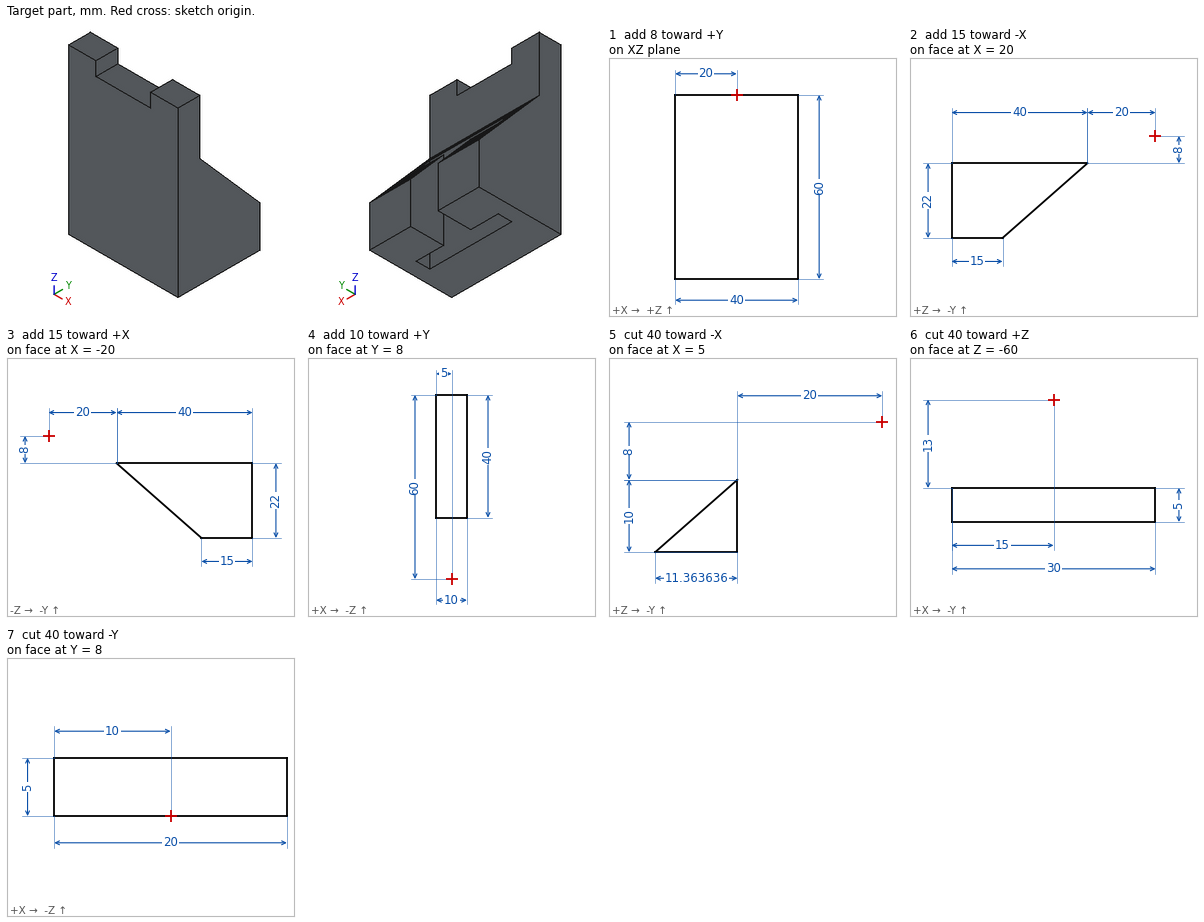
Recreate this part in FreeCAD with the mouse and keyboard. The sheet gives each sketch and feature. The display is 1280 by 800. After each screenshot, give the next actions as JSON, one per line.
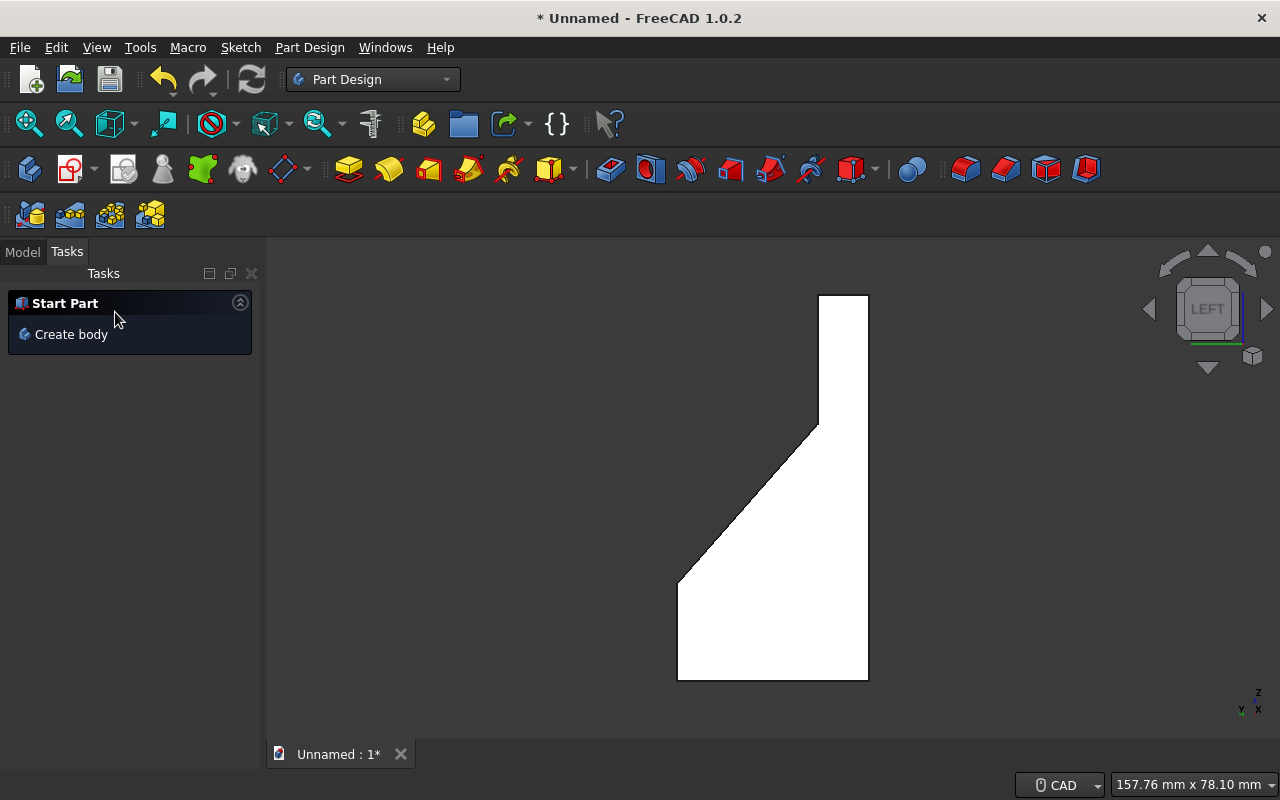
{"action": "key", "text": "4"}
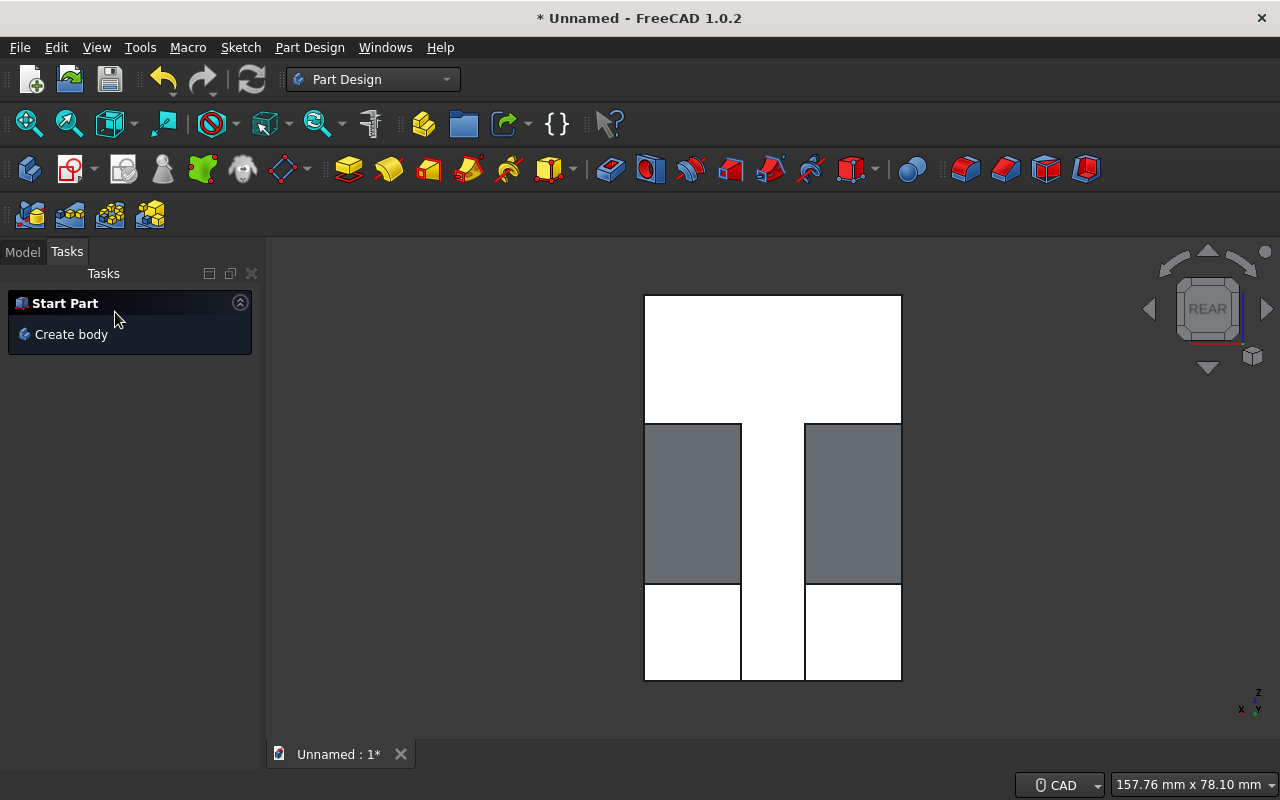
{"action": "left_click", "coordinate": [773, 377]}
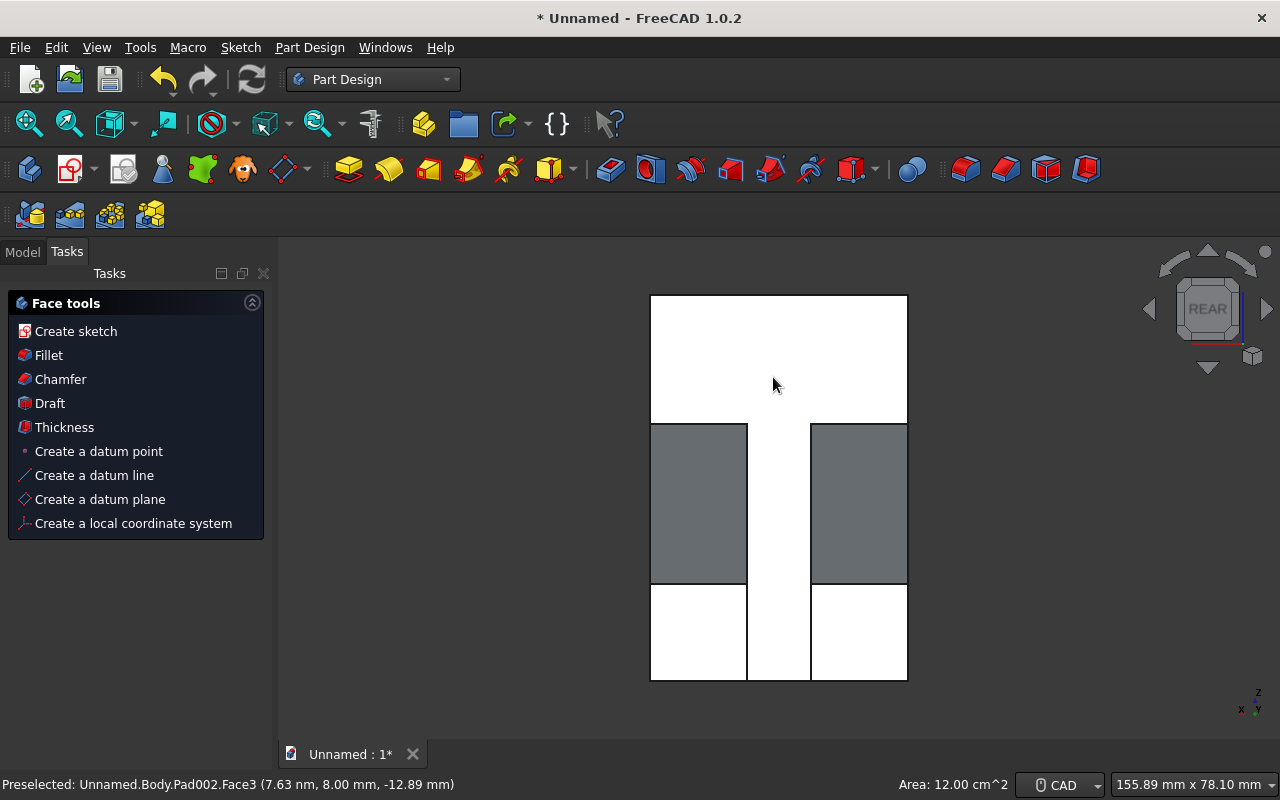
{"action": "left_click", "coordinate": [70, 170]}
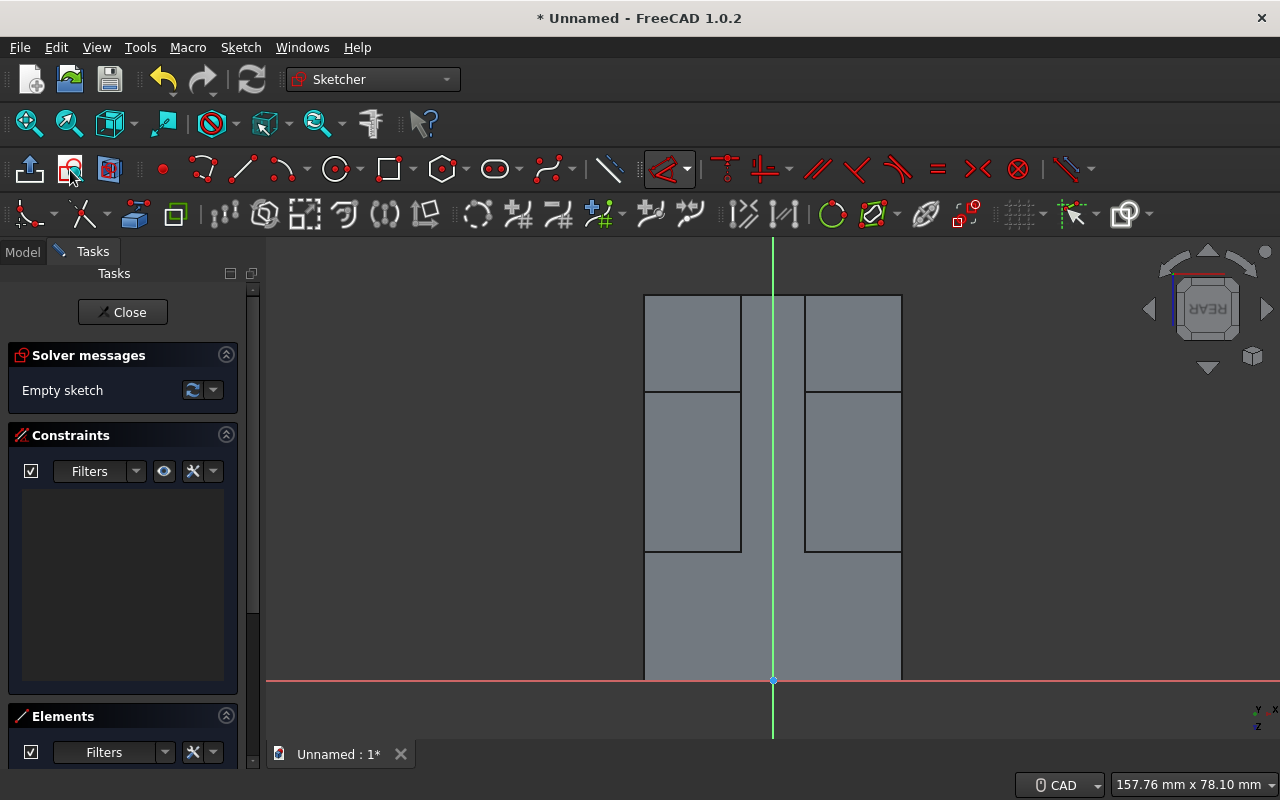
{"action": "left_click", "coordinate": [110, 170]}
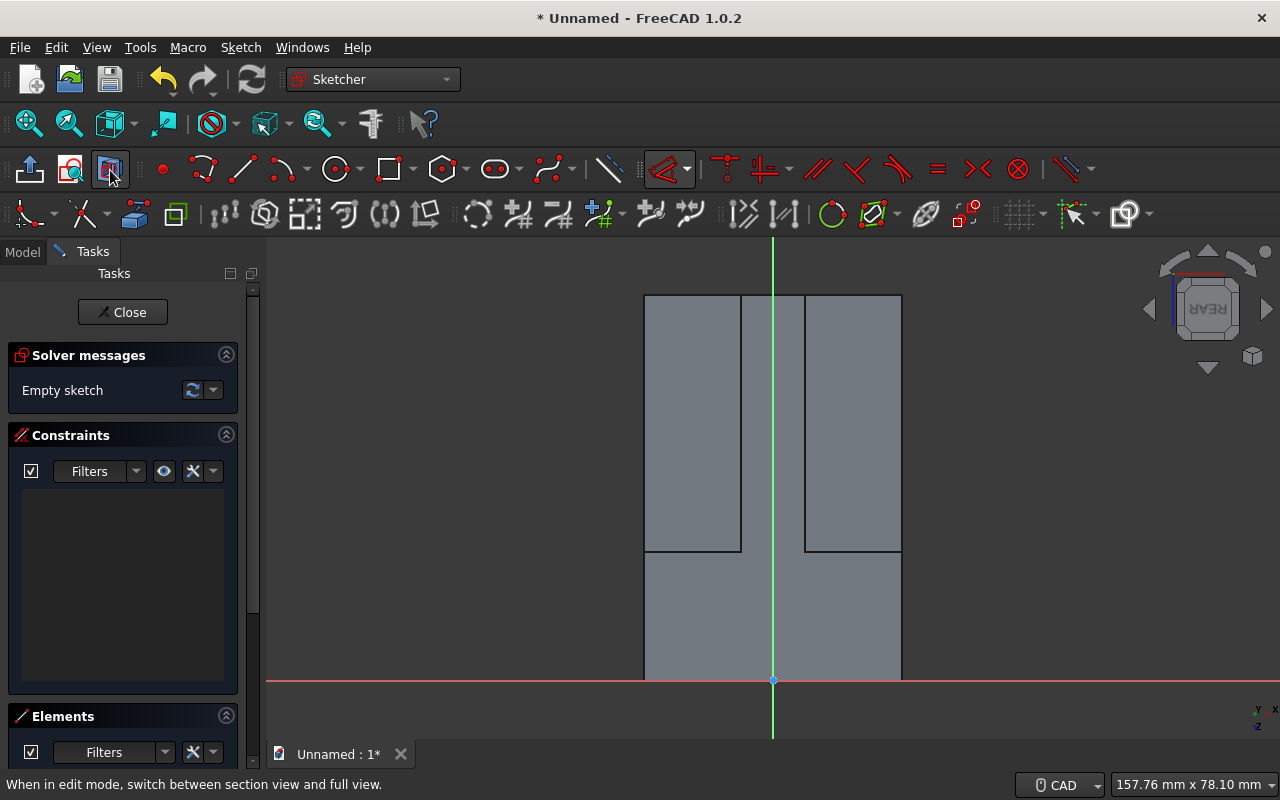
{"action": "left_click", "coordinate": [390, 170]}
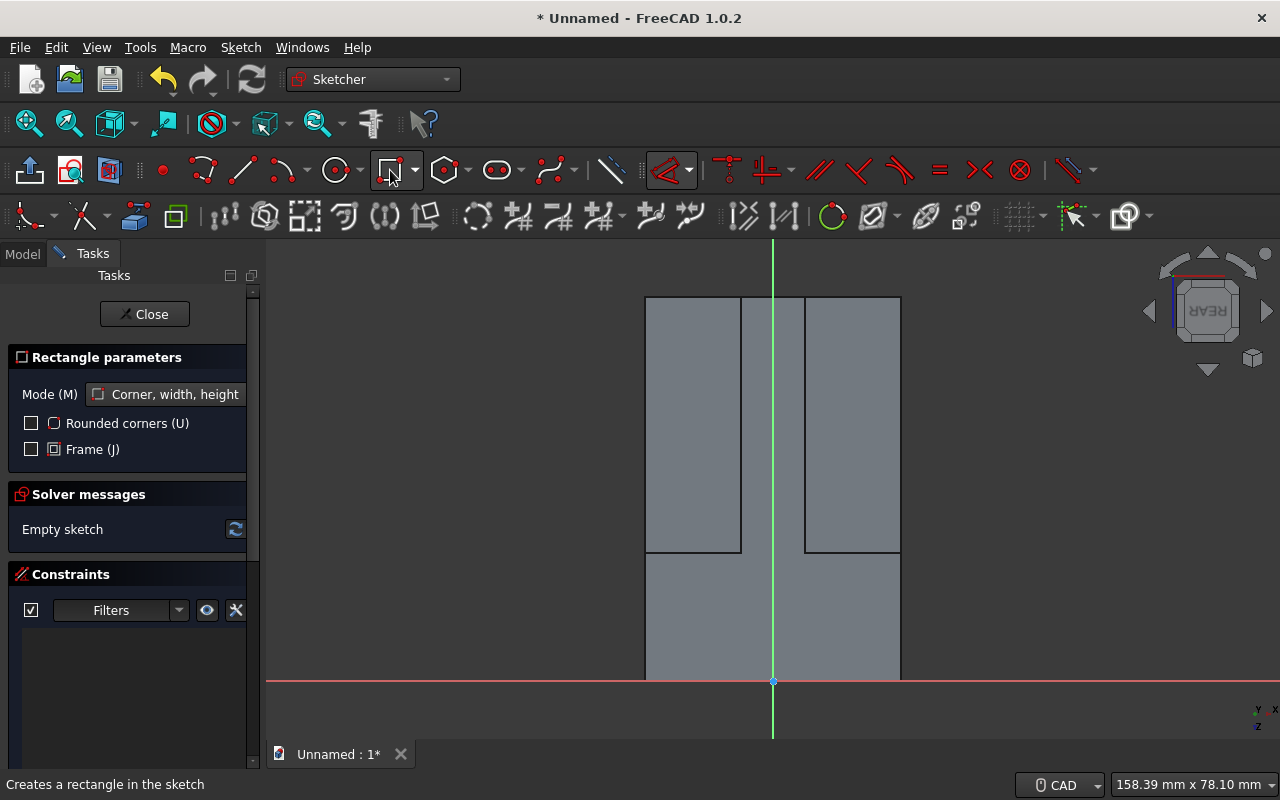
{"action": "left_click", "coordinate": [741, 297]}
{"action": "mouse_move", "coordinate": [805, 553]}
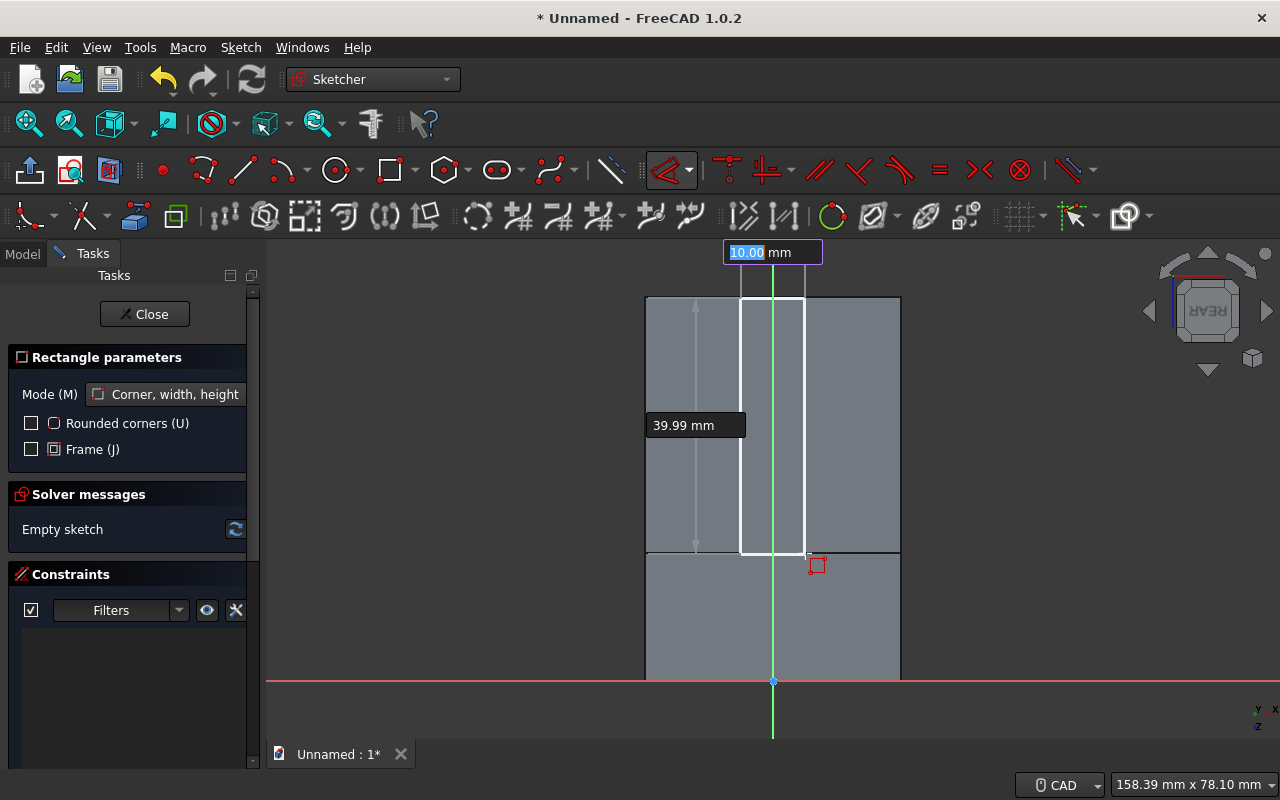
{"action": "type", "text": "10"}
{"action": "key", "text": "Tab"}
{"action": "type", "text": "40"}
{"action": "key", "text": "Return"}
{"action": "key", "text": "Escape"}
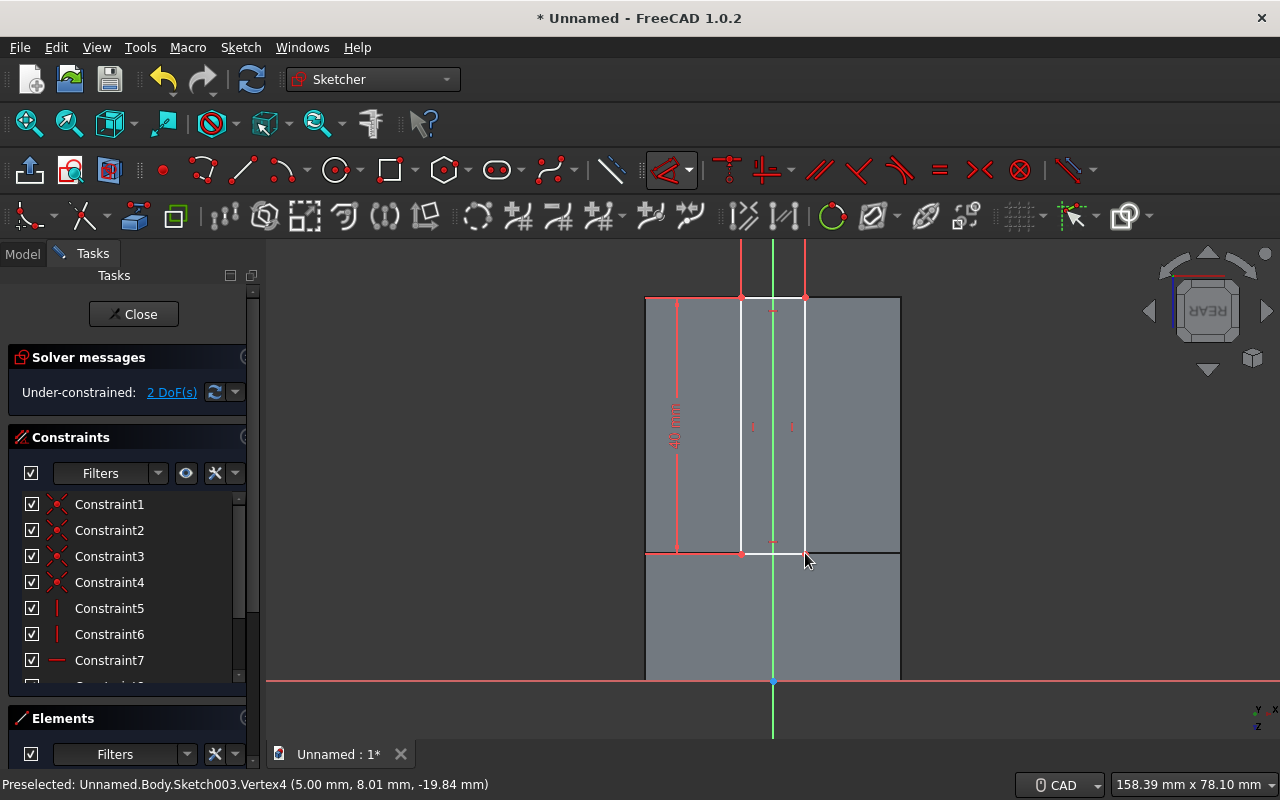
{"action": "scroll", "coordinate": [741, 298], "scroll_direction": "up", "scroll_amount": 2}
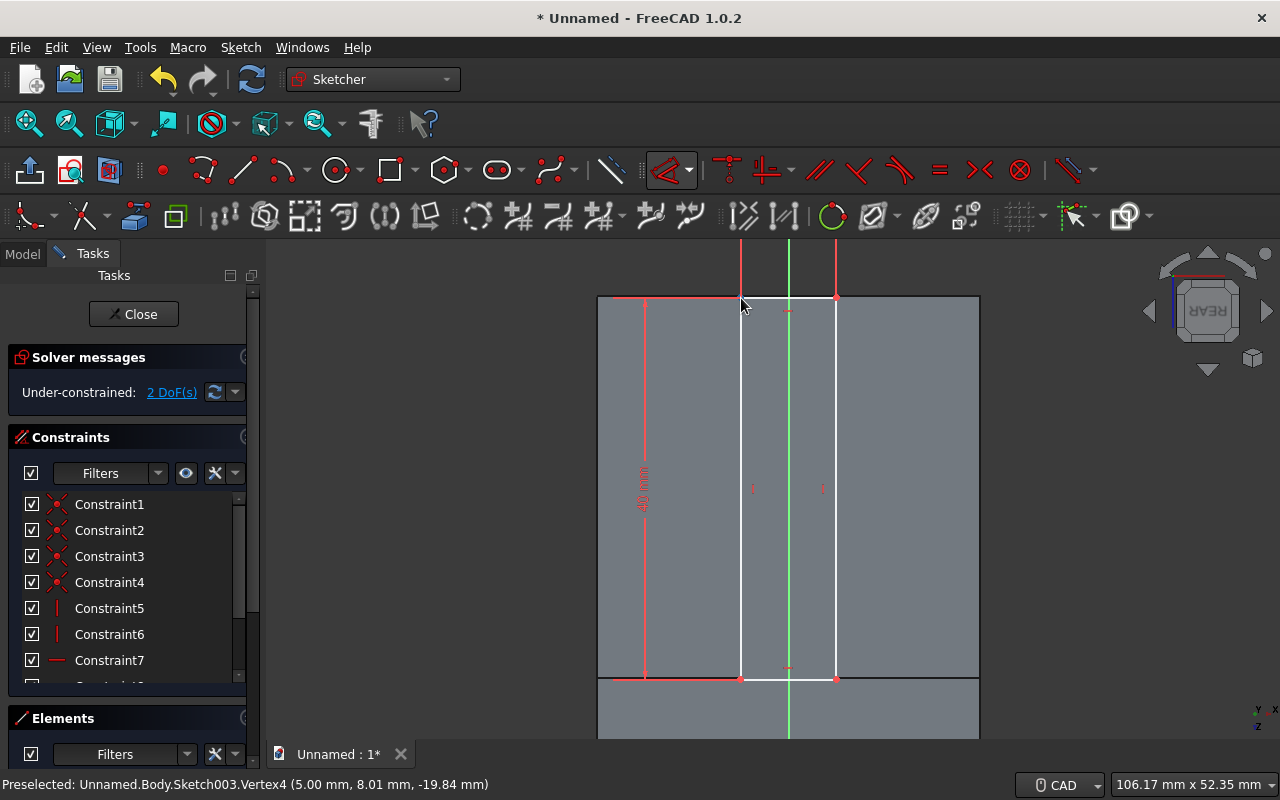
{"action": "left_click", "coordinate": [741, 298]}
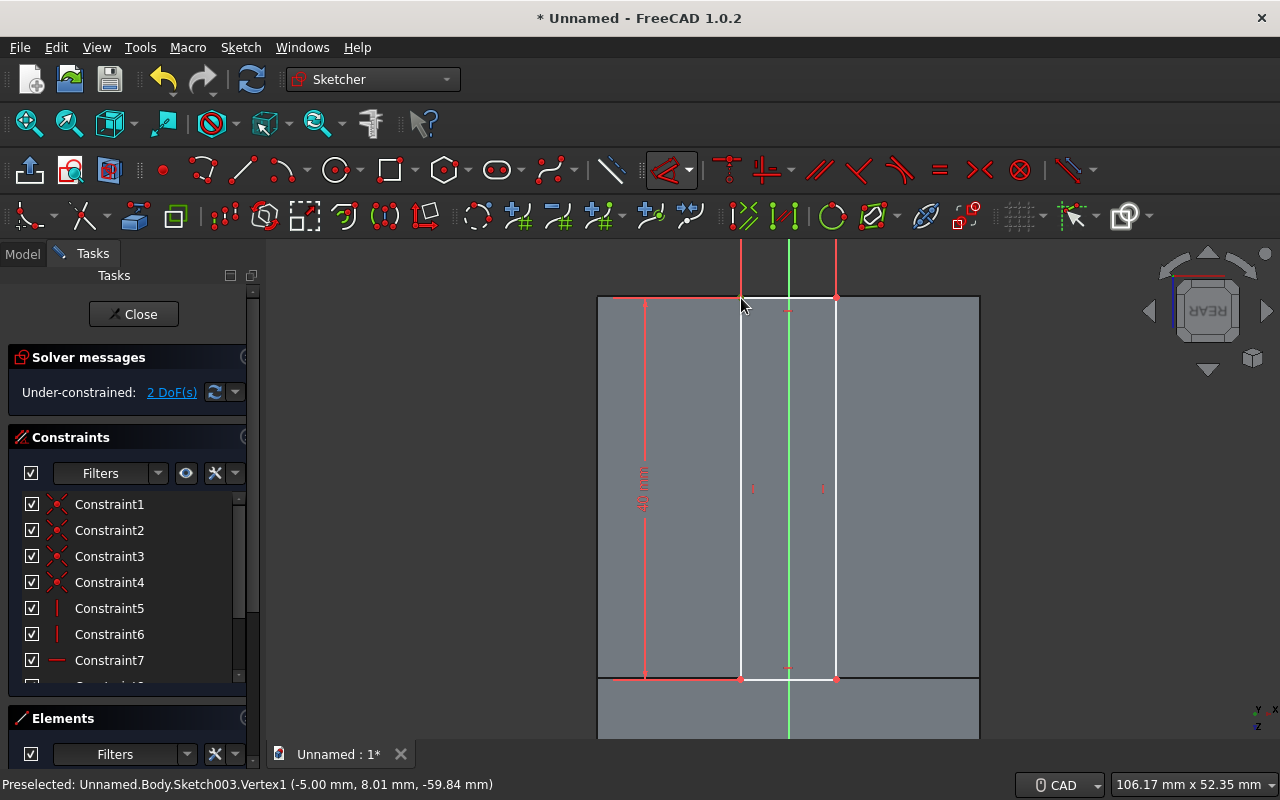
{"action": "left_click", "coordinate": [692, 170]}